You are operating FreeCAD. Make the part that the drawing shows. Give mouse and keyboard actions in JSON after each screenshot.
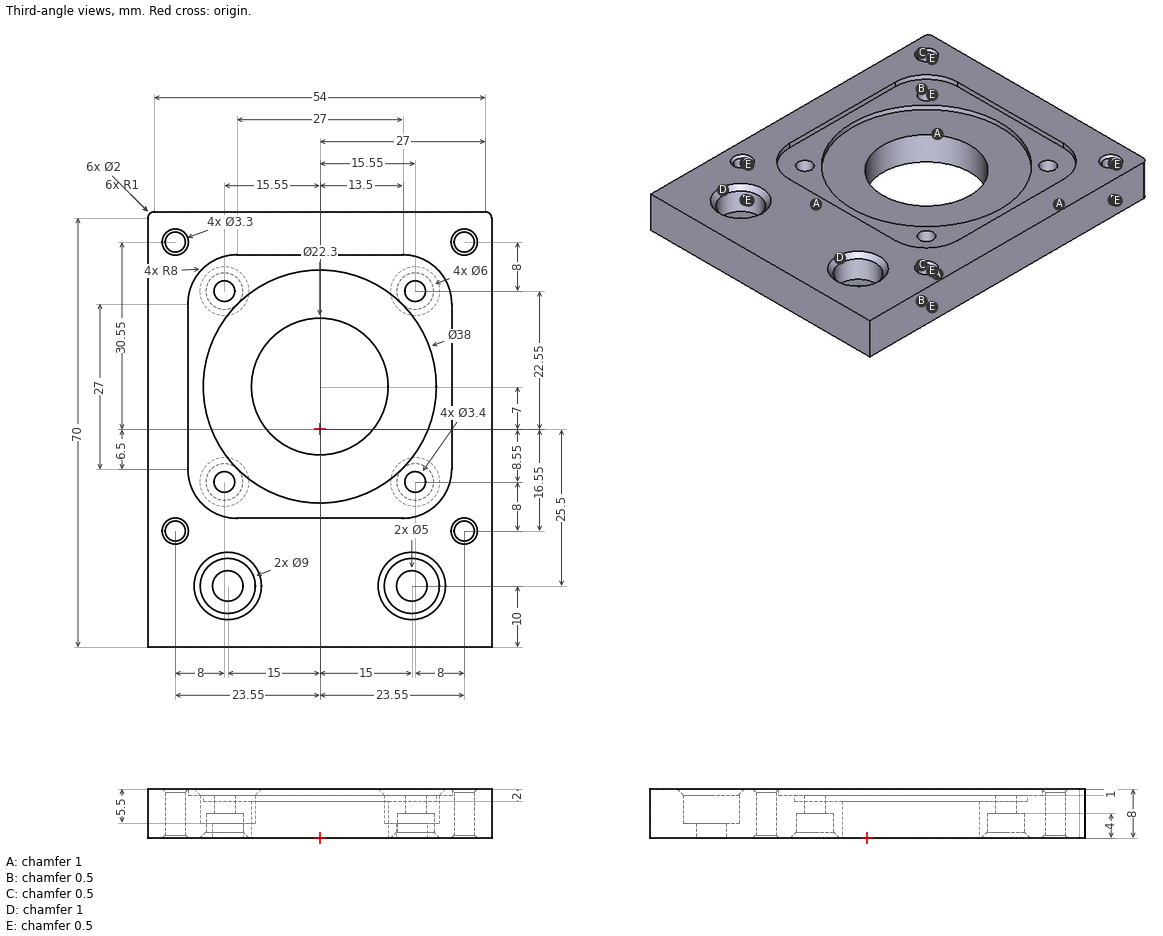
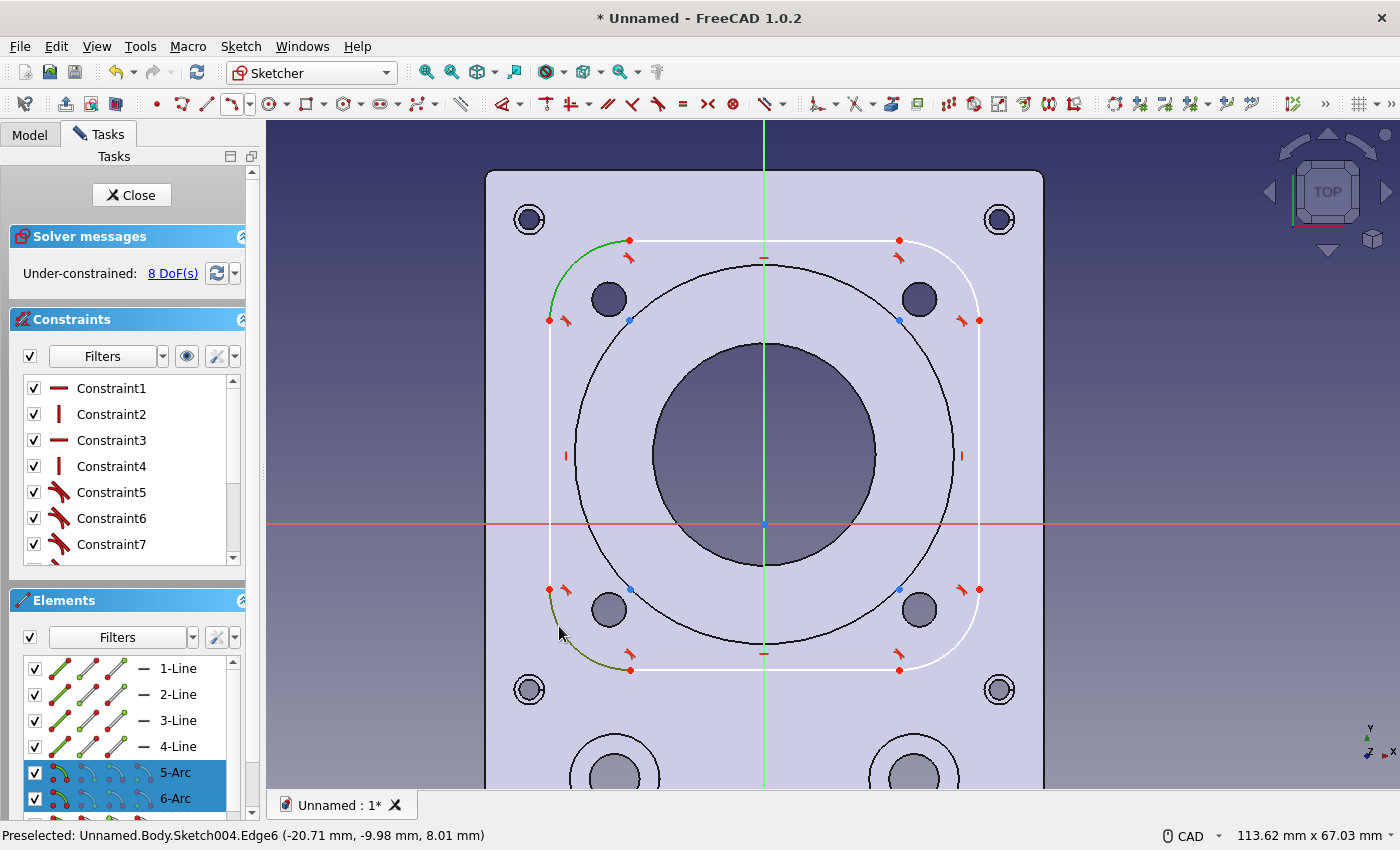
{"action": "left_click", "coordinate": [935, 661]}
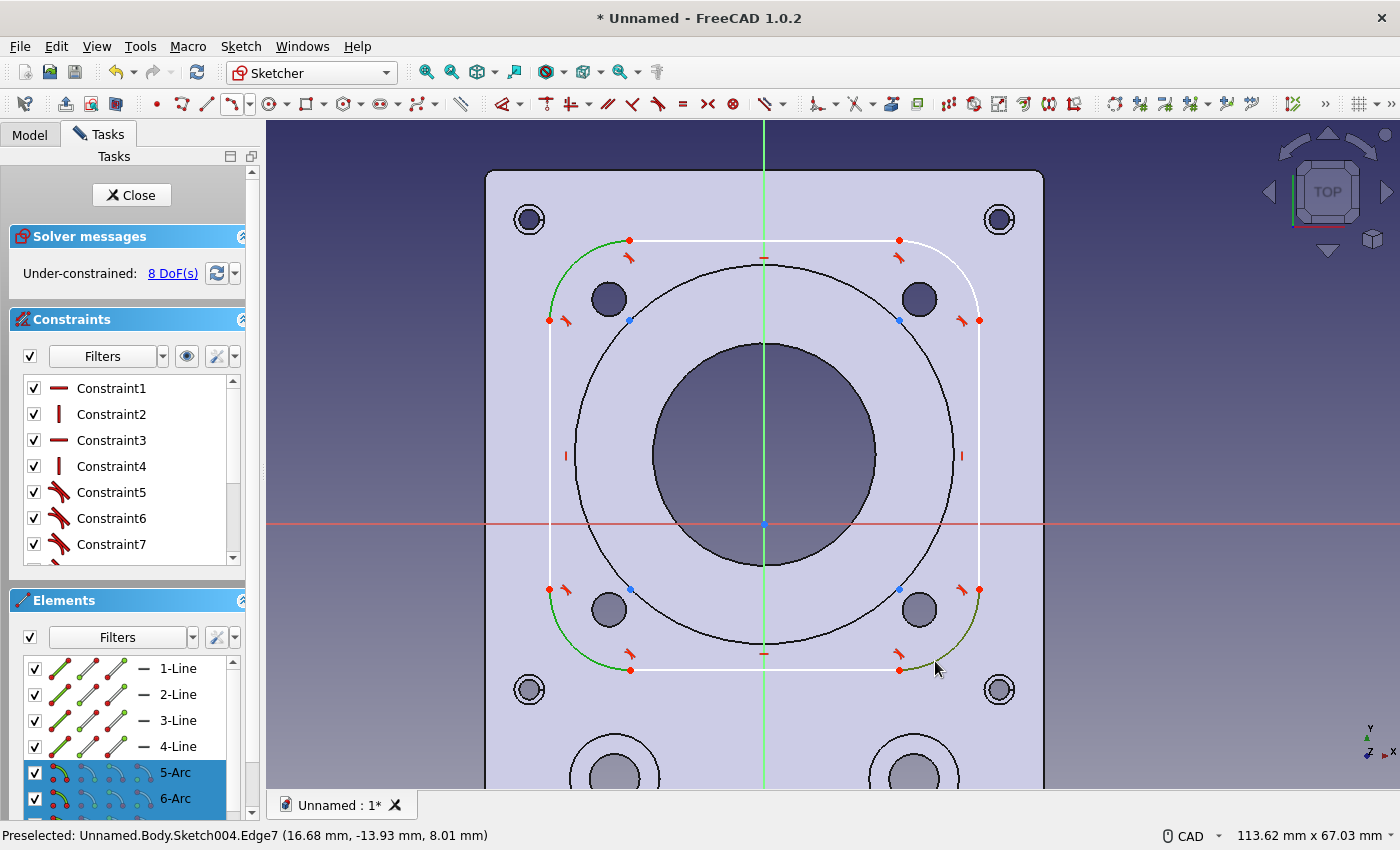
{"action": "left_click", "coordinate": [970, 285]}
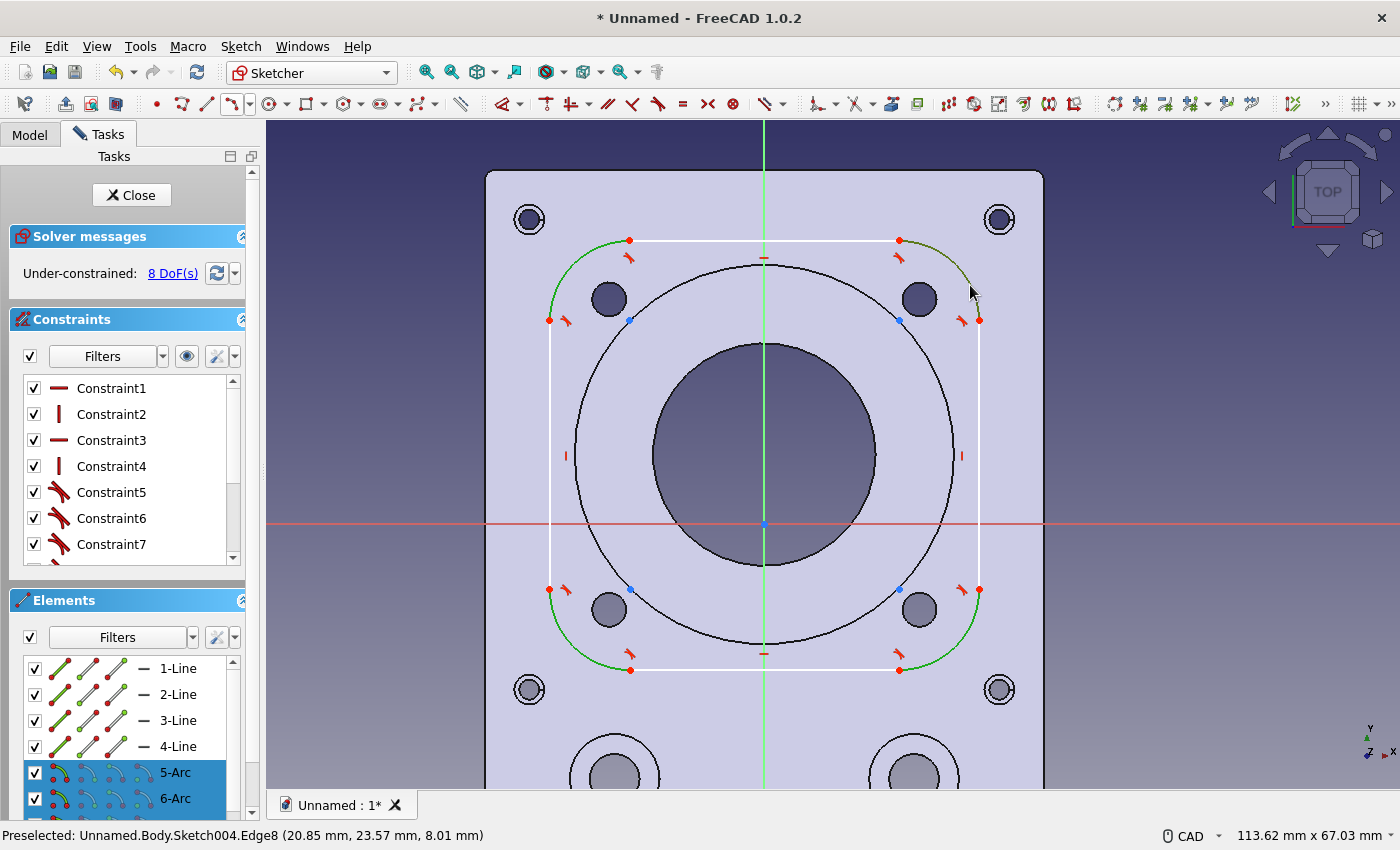
{"action": "left_click", "coordinate": [683, 104]}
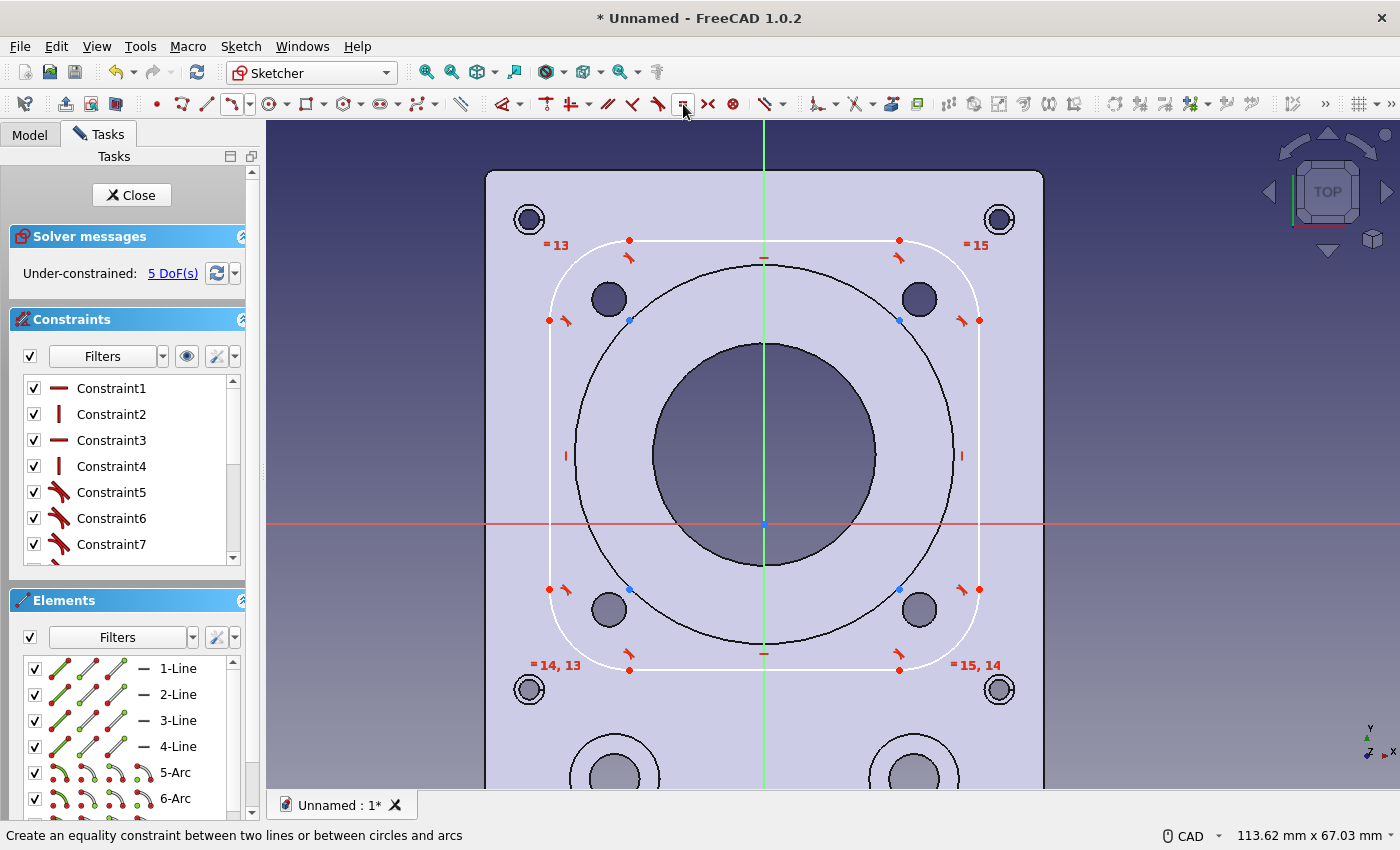
{"action": "key", "text": "d"}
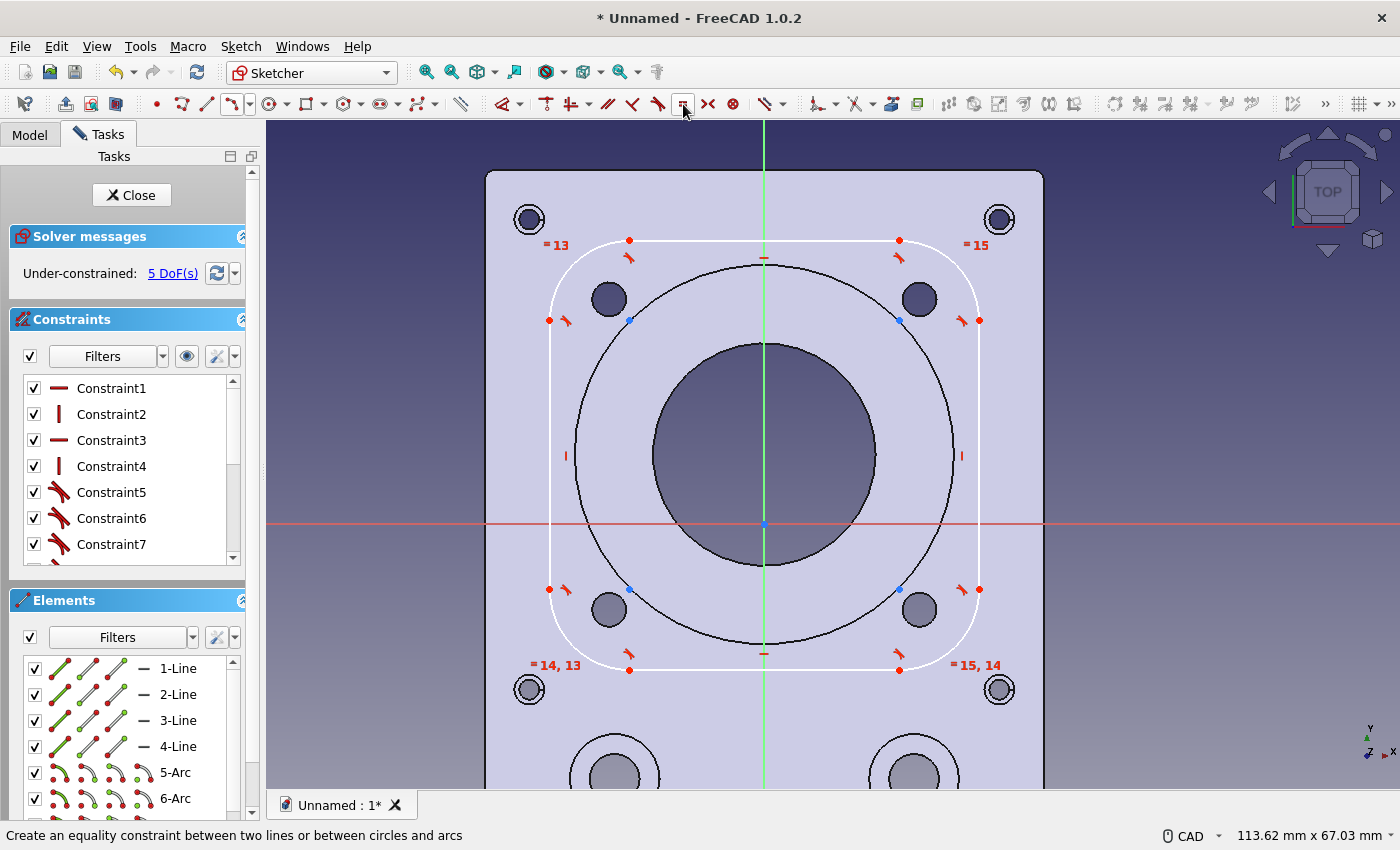
{"action": "left_click", "coordinate": [594, 250]}
{"action": "left_click", "coordinate": [580, 221]}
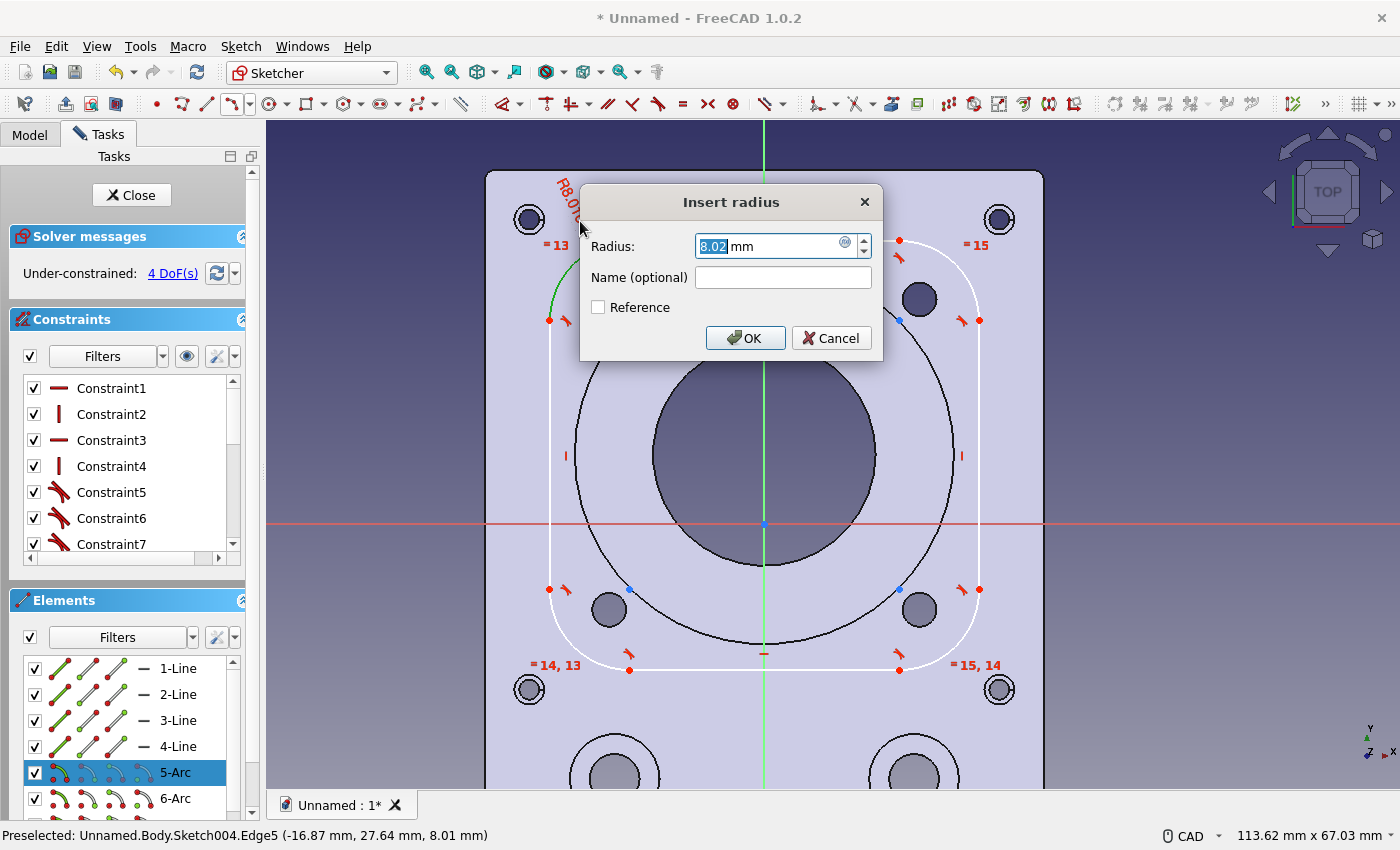
{"action": "type", "text": "8"}
{"action": "key", "text": "Return"}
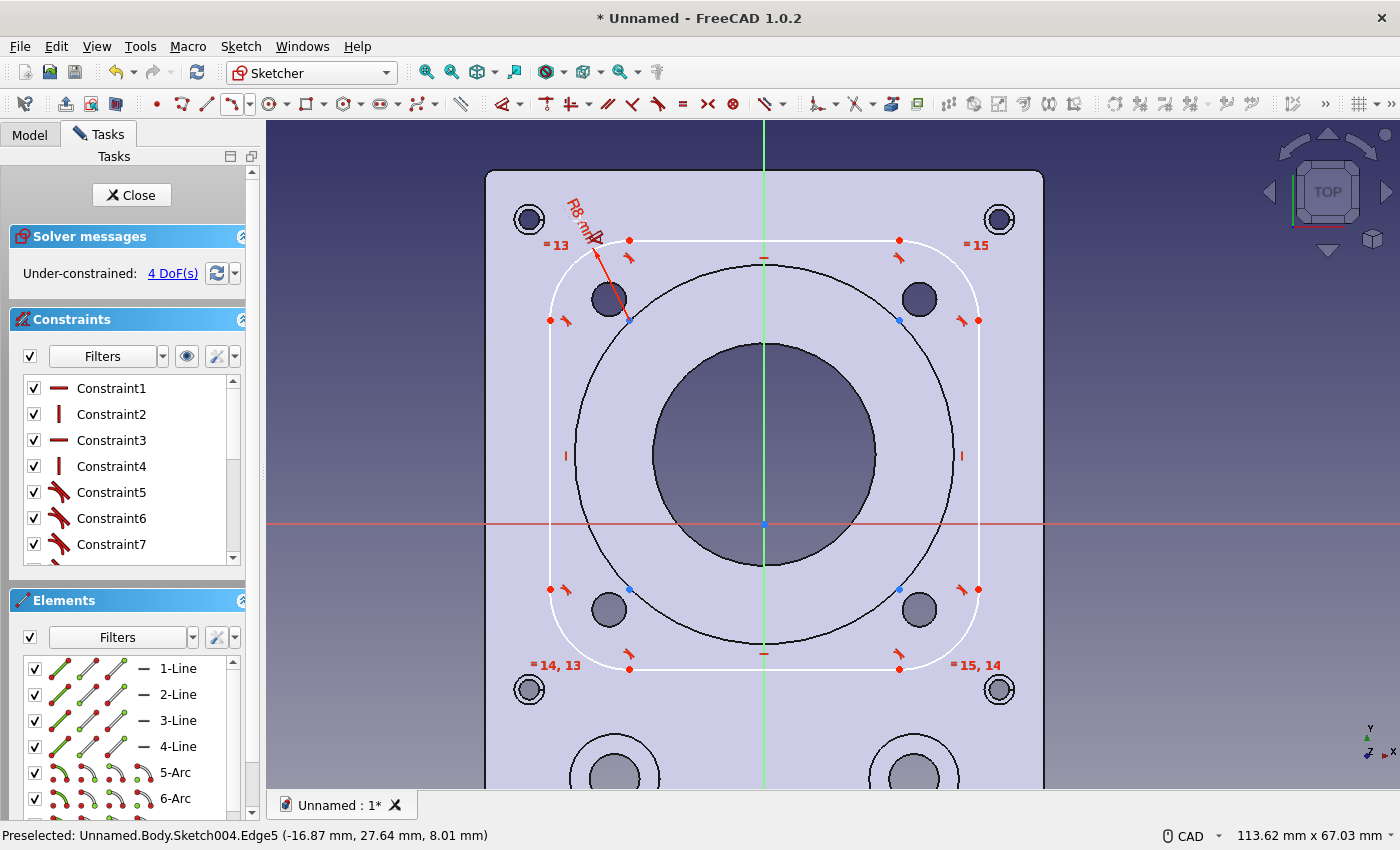
{"action": "left_click", "coordinate": [818, 241]}
{"action": "left_click", "coordinate": [703, 207]}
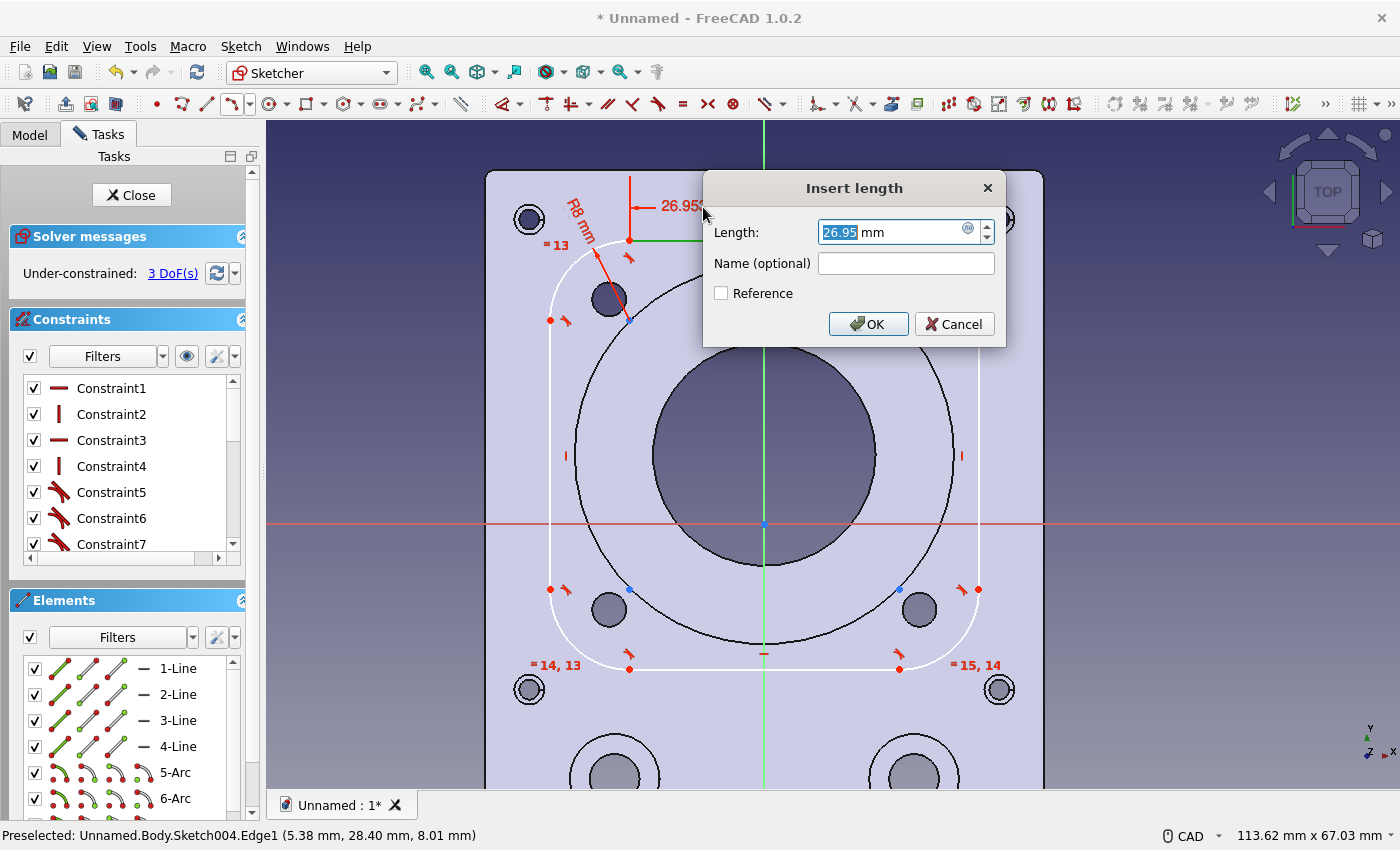
{"action": "type", "text": "27"}
{"action": "key", "text": "Return"}